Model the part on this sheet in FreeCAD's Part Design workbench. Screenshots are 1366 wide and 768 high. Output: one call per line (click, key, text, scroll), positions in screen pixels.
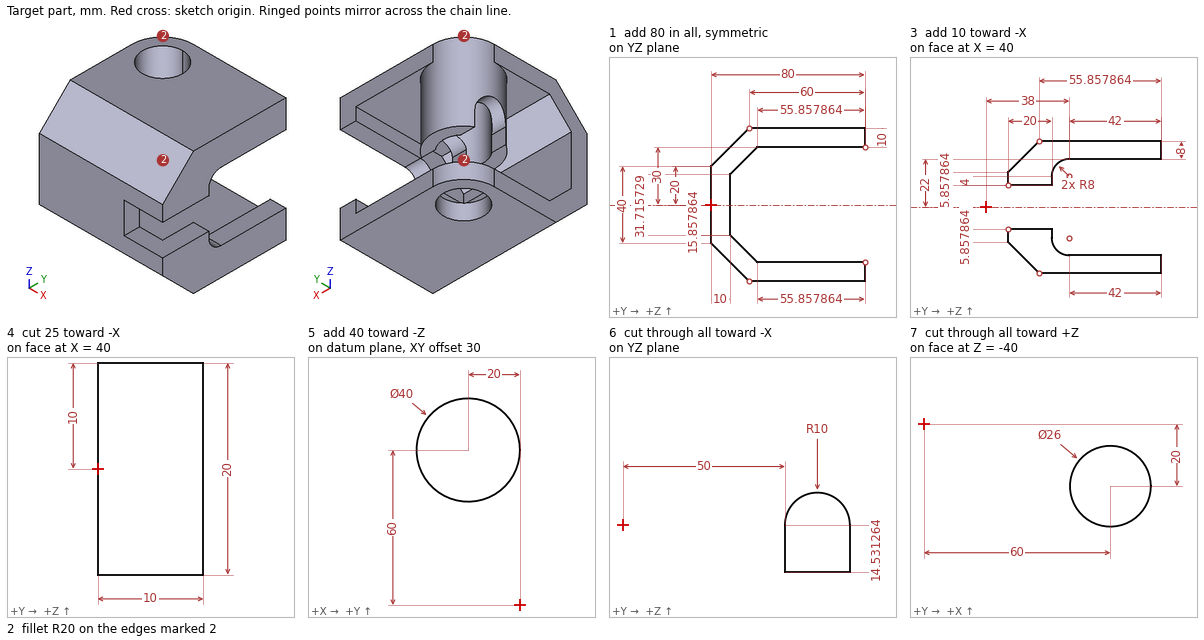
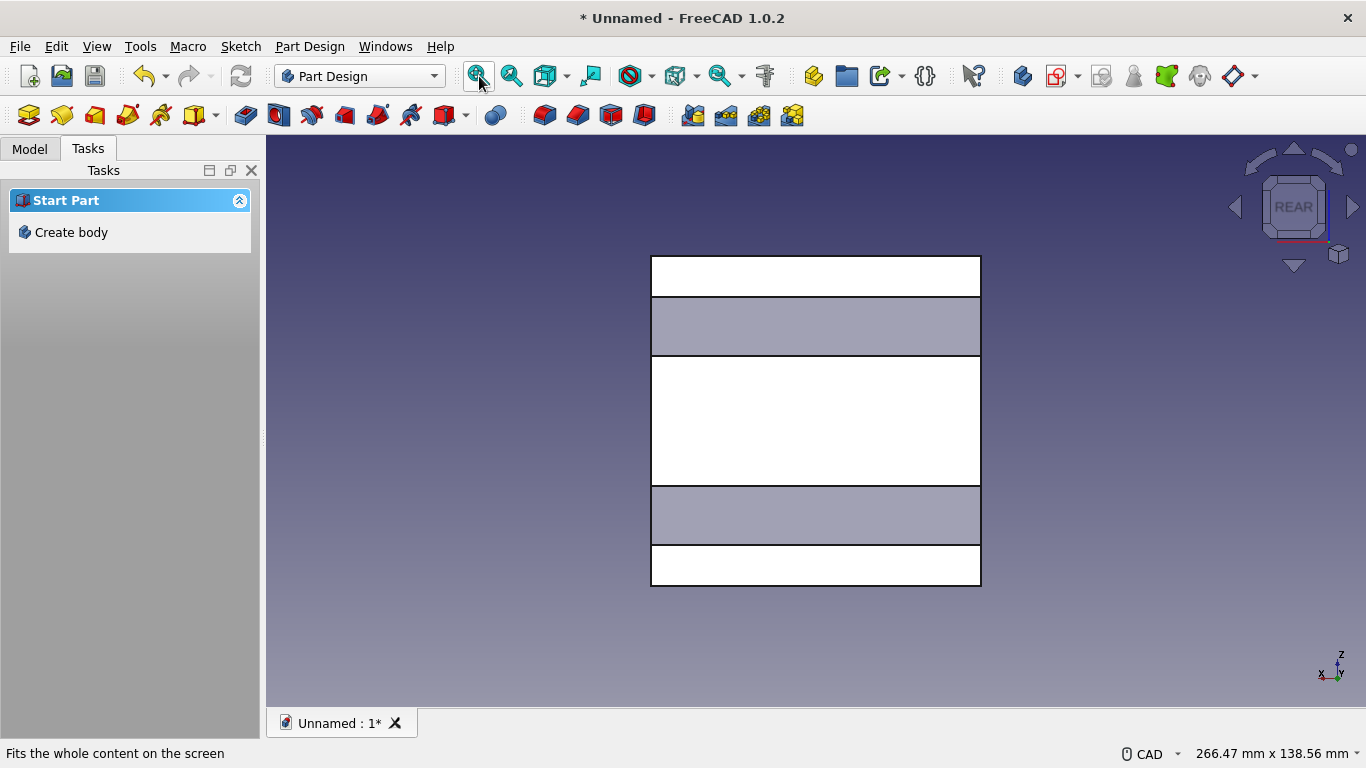
click(981, 276)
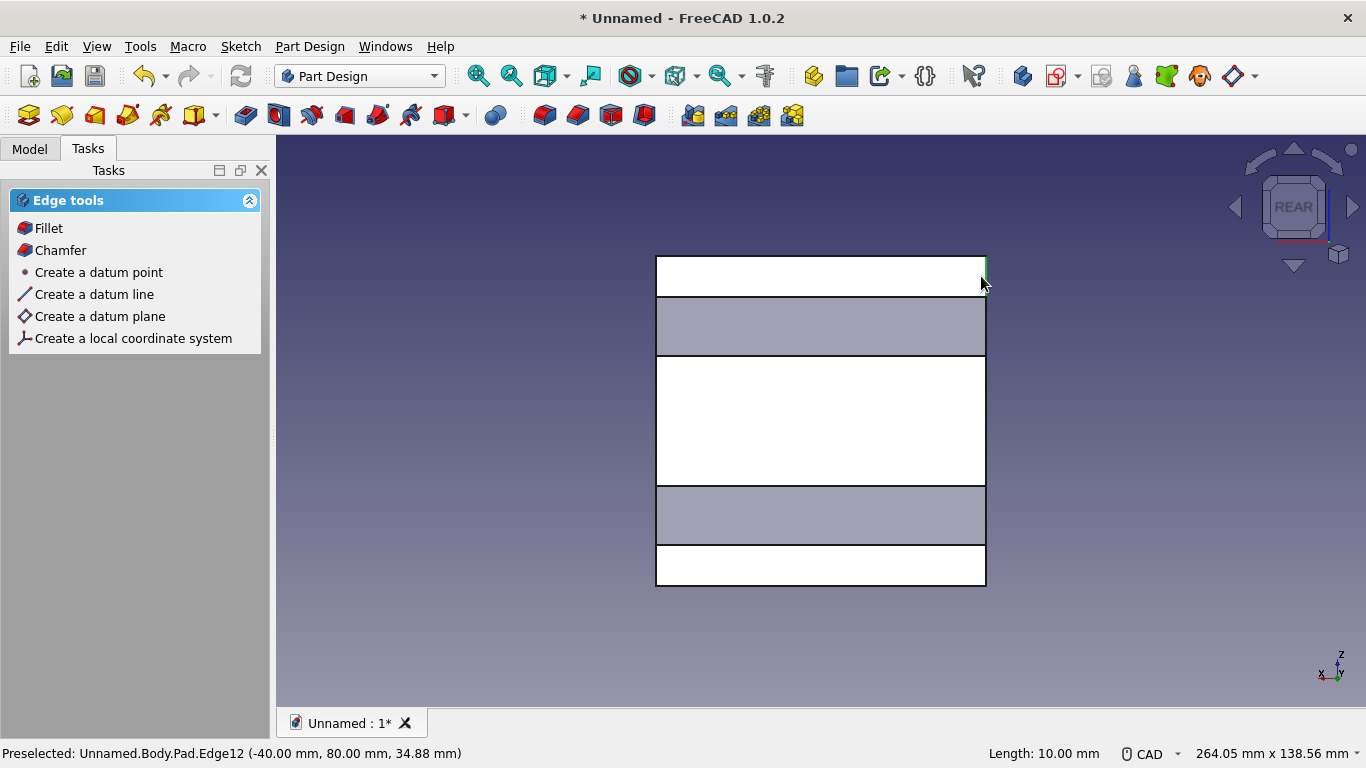
click(986, 564, ctrl)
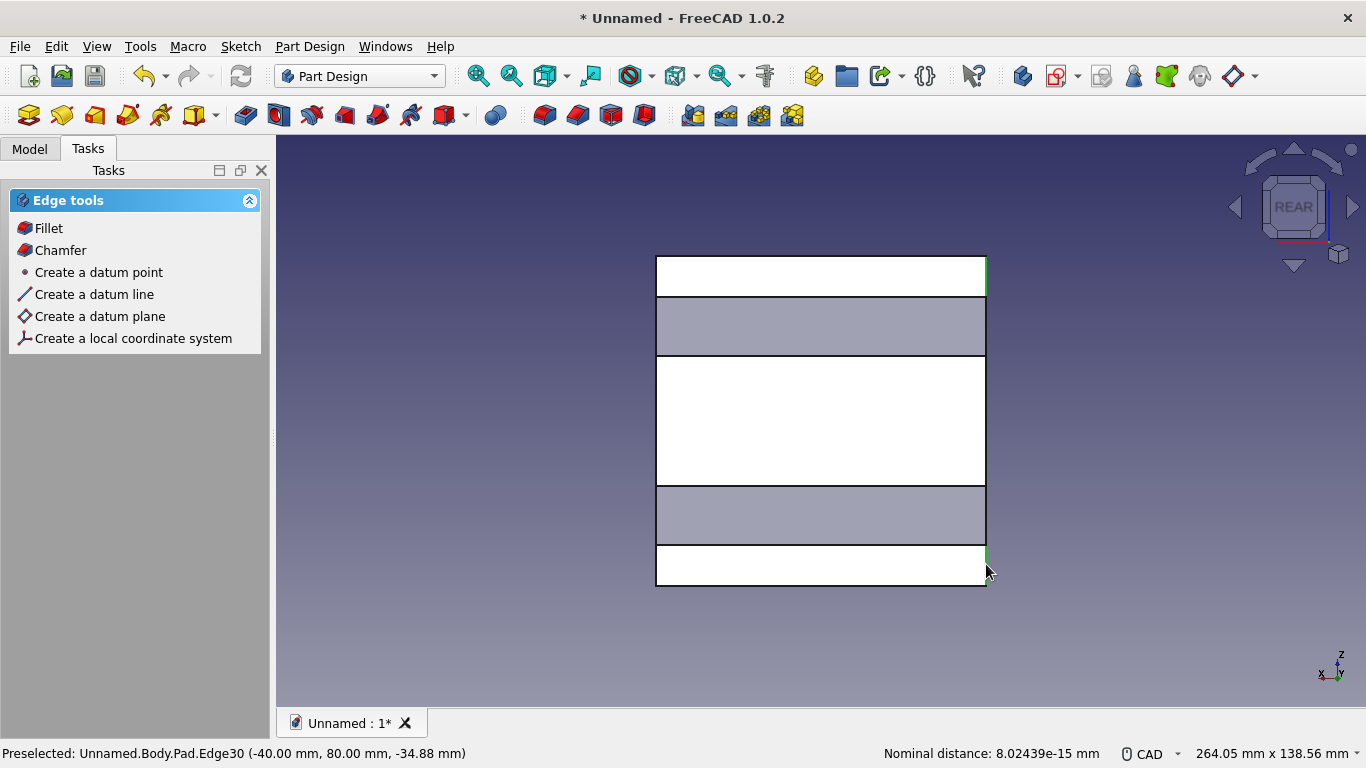
click(545, 116)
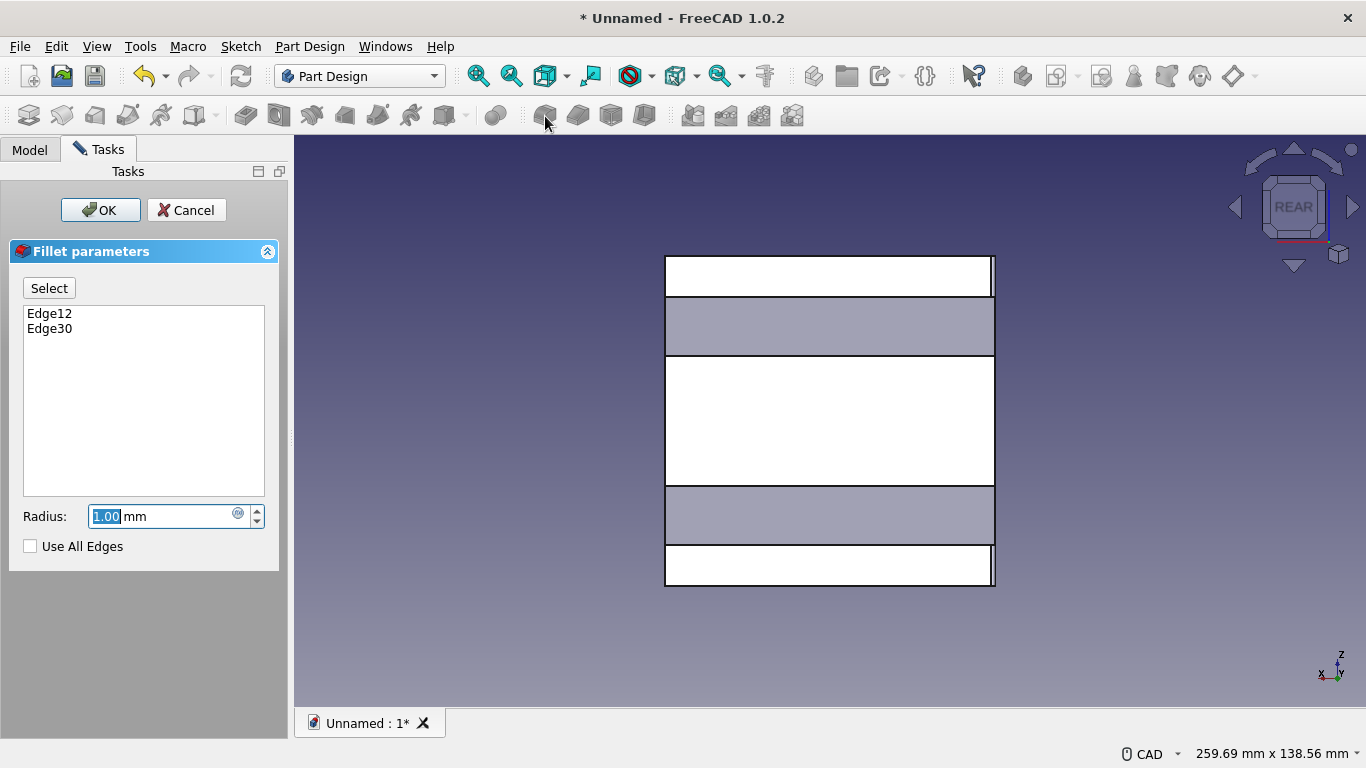
text(20)
key(Tab)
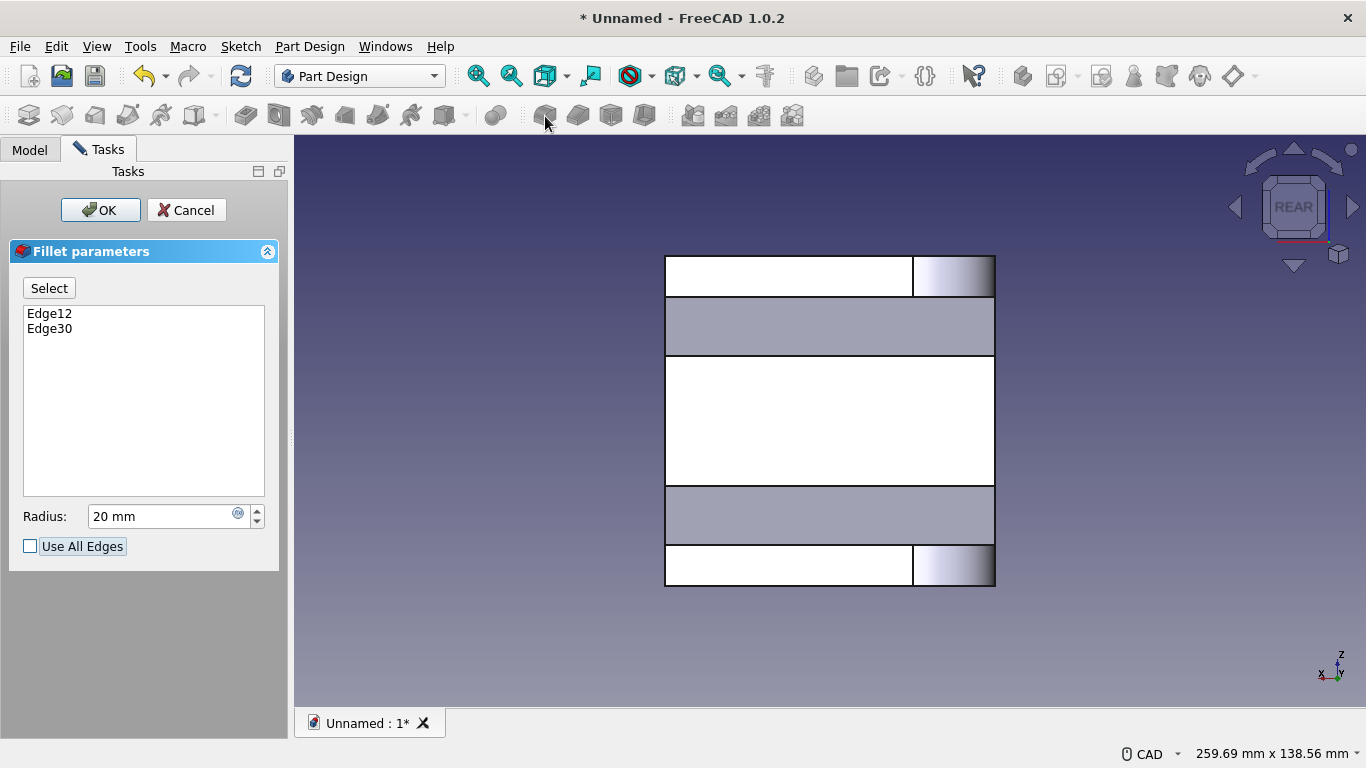
click(101, 210)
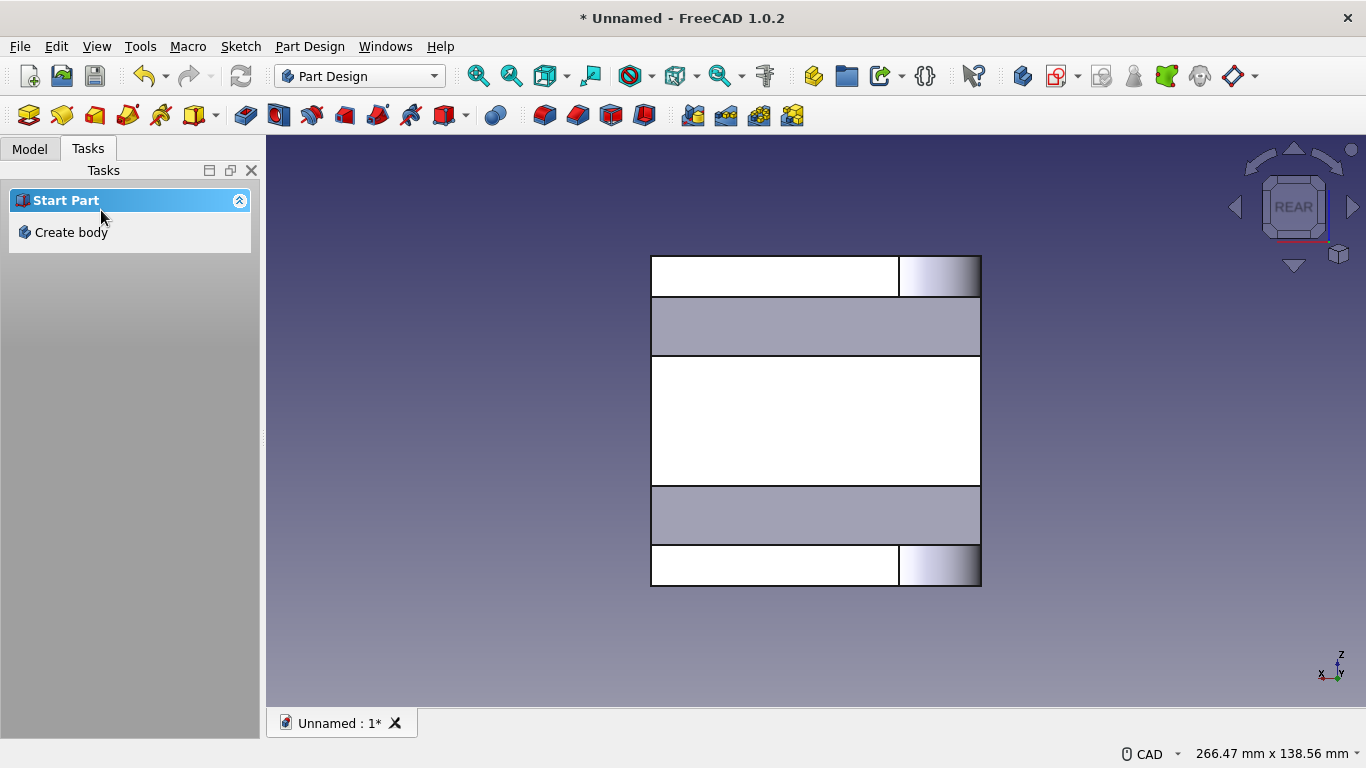
key(0)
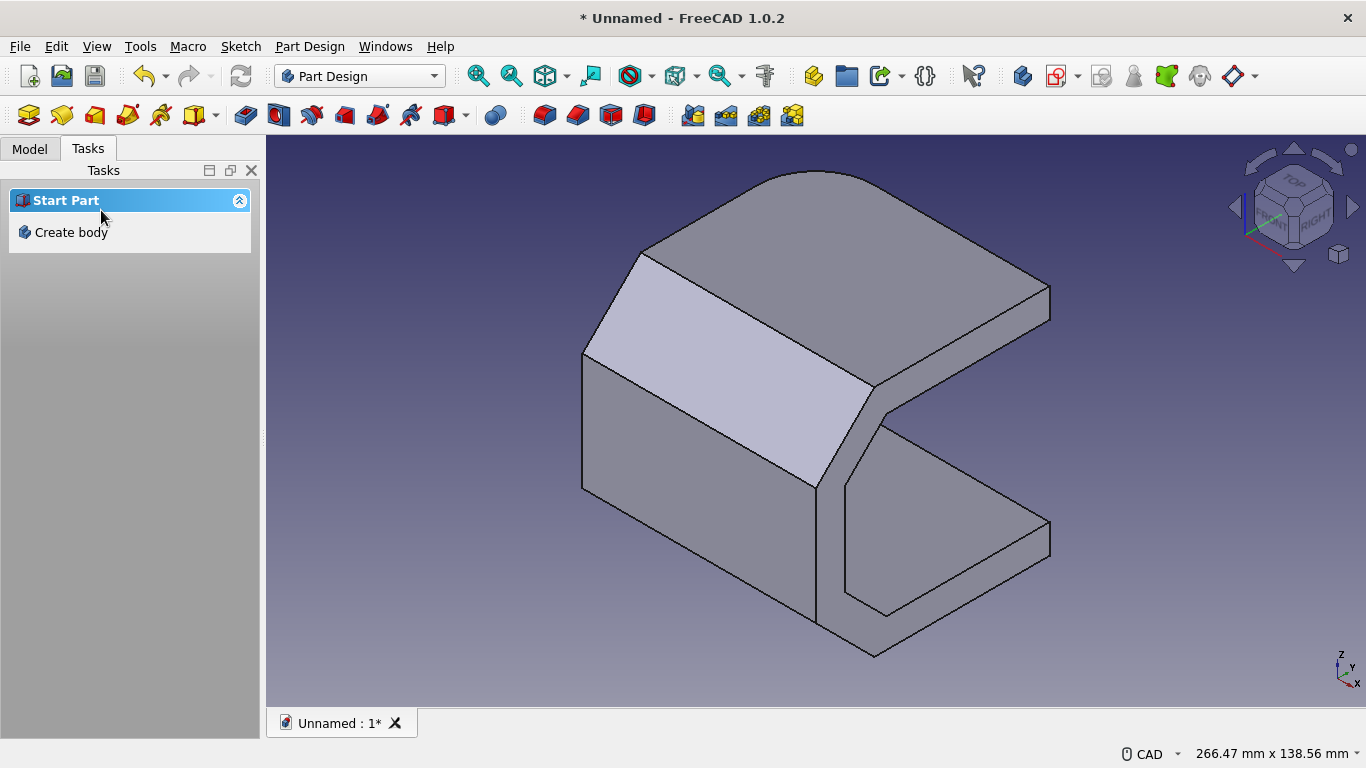
click(1033, 314)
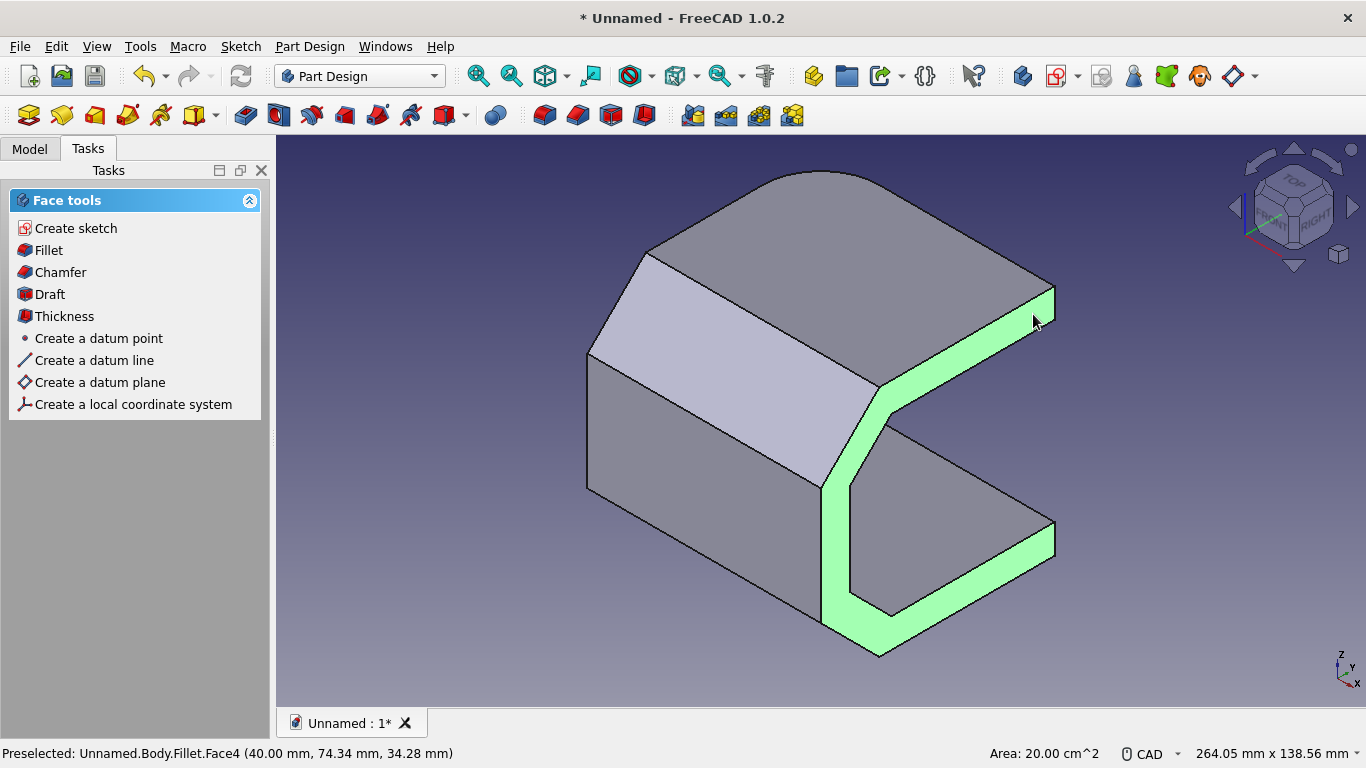
click(1056, 76)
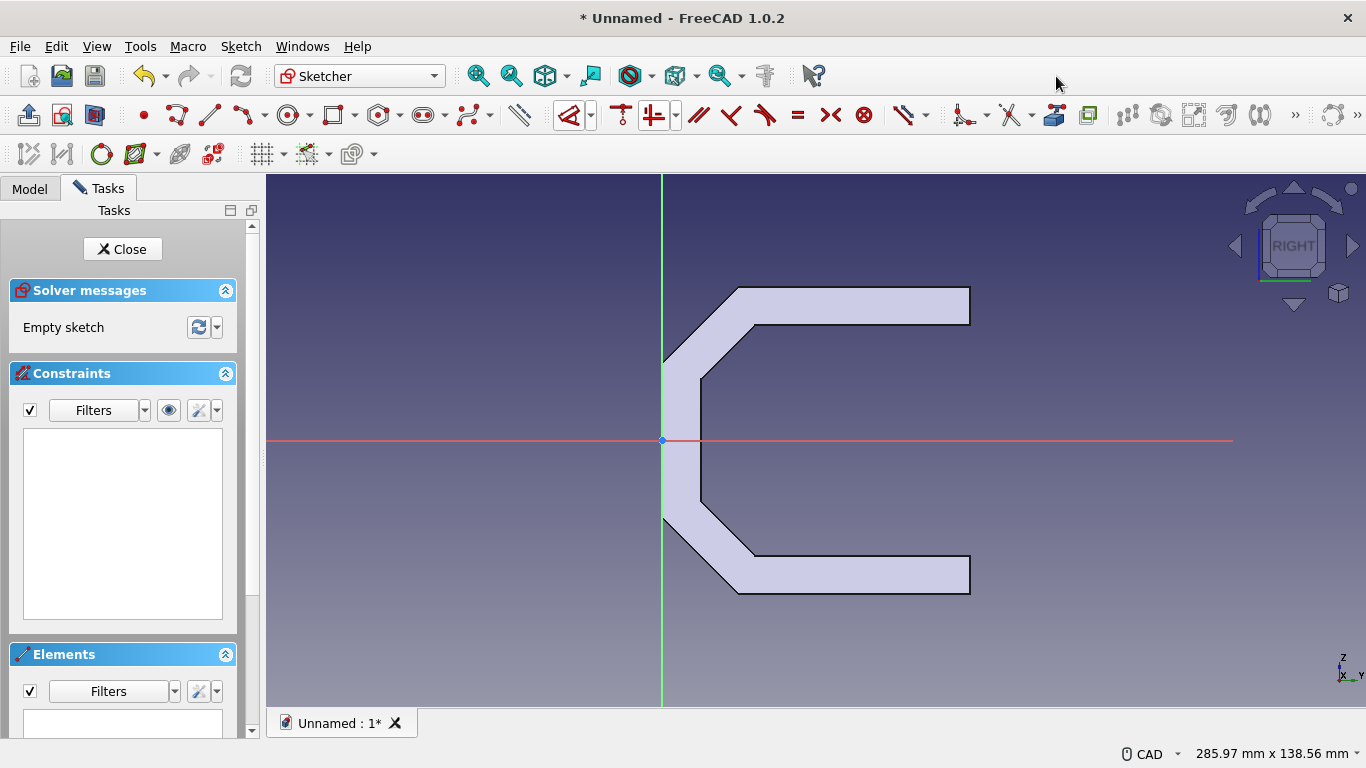
scroll(955, 440, up, 2)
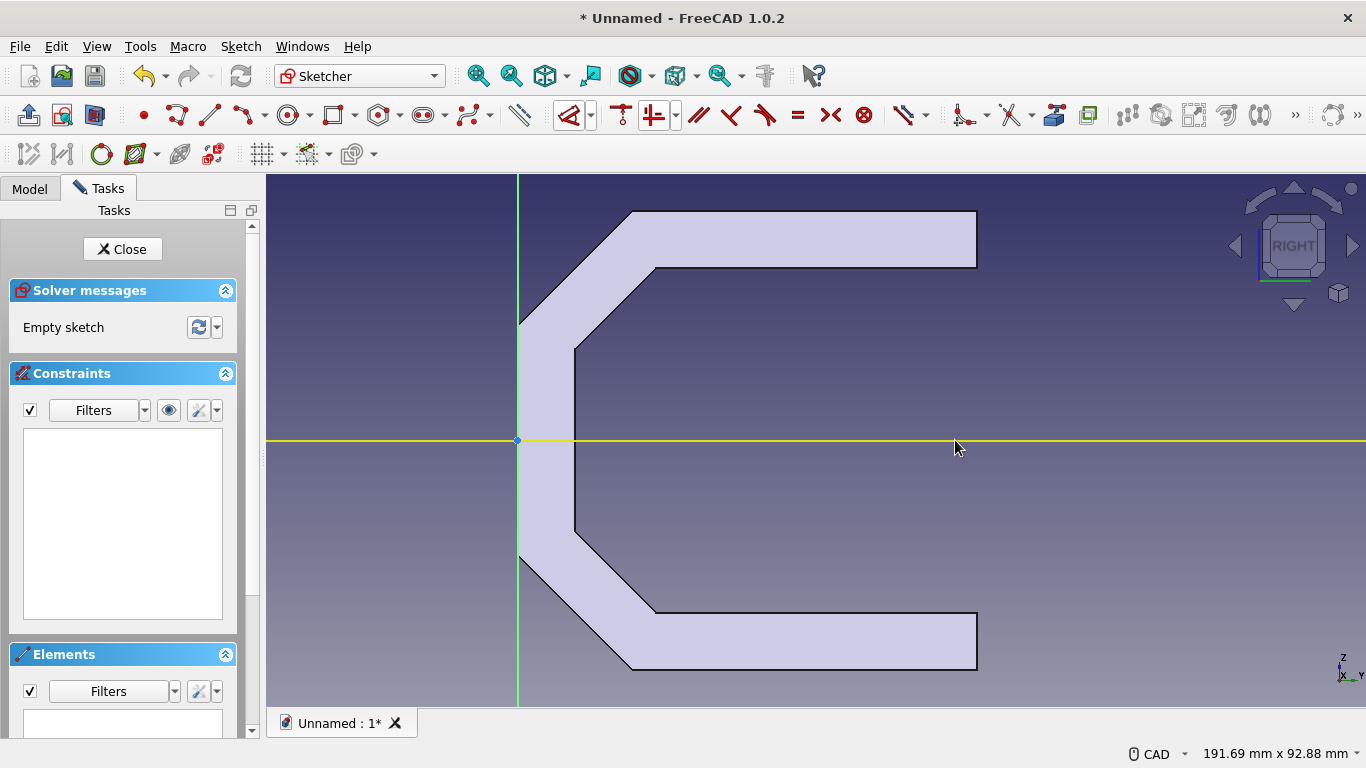
click(177, 116)